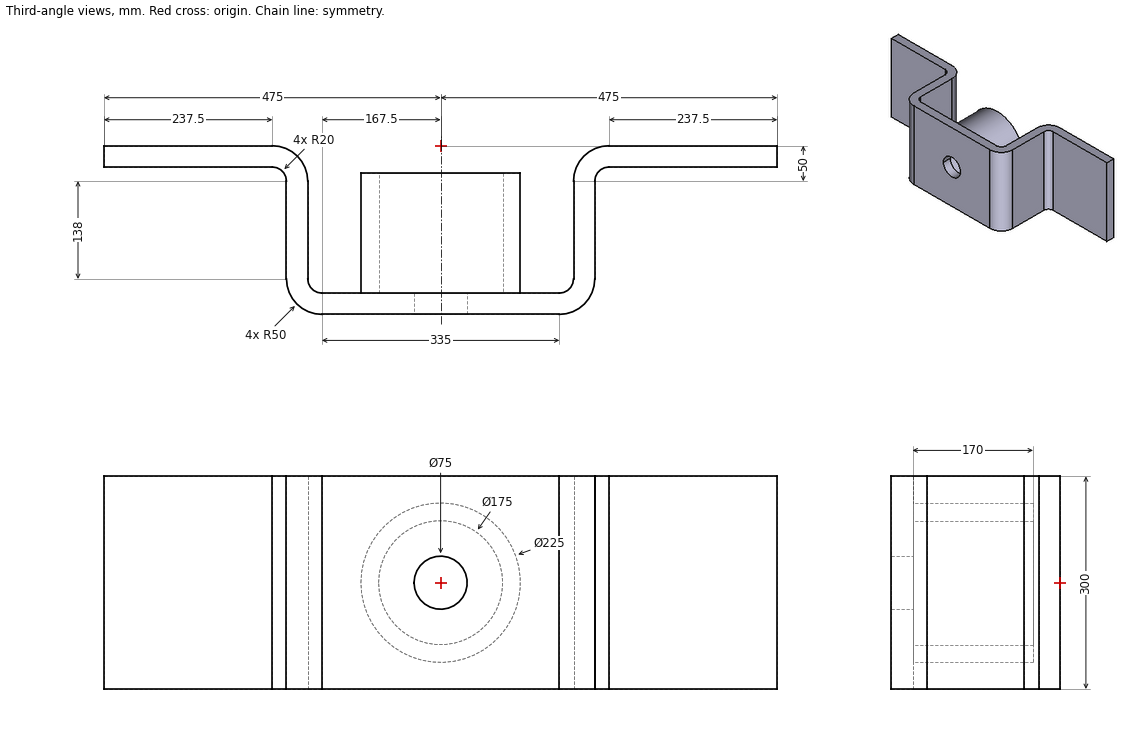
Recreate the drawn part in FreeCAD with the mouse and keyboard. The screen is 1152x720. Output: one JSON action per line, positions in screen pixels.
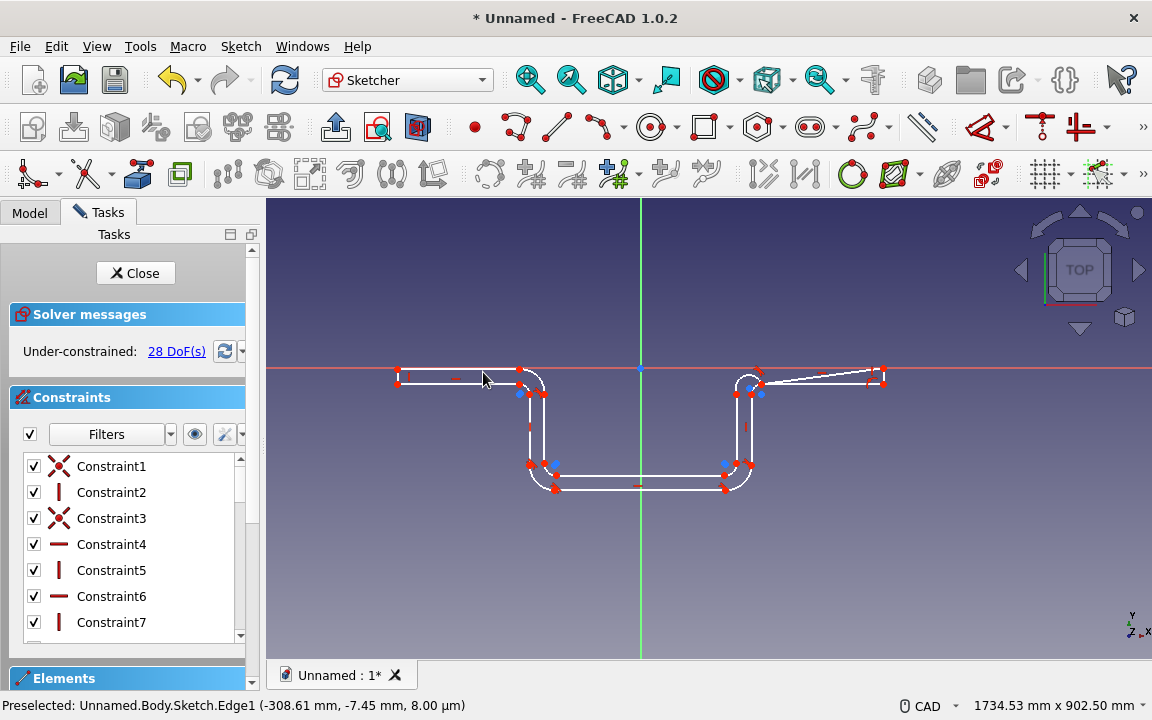
{"action": "scroll", "coordinate": [847, 373], "scroll_direction": "up", "scroll_amount": 6}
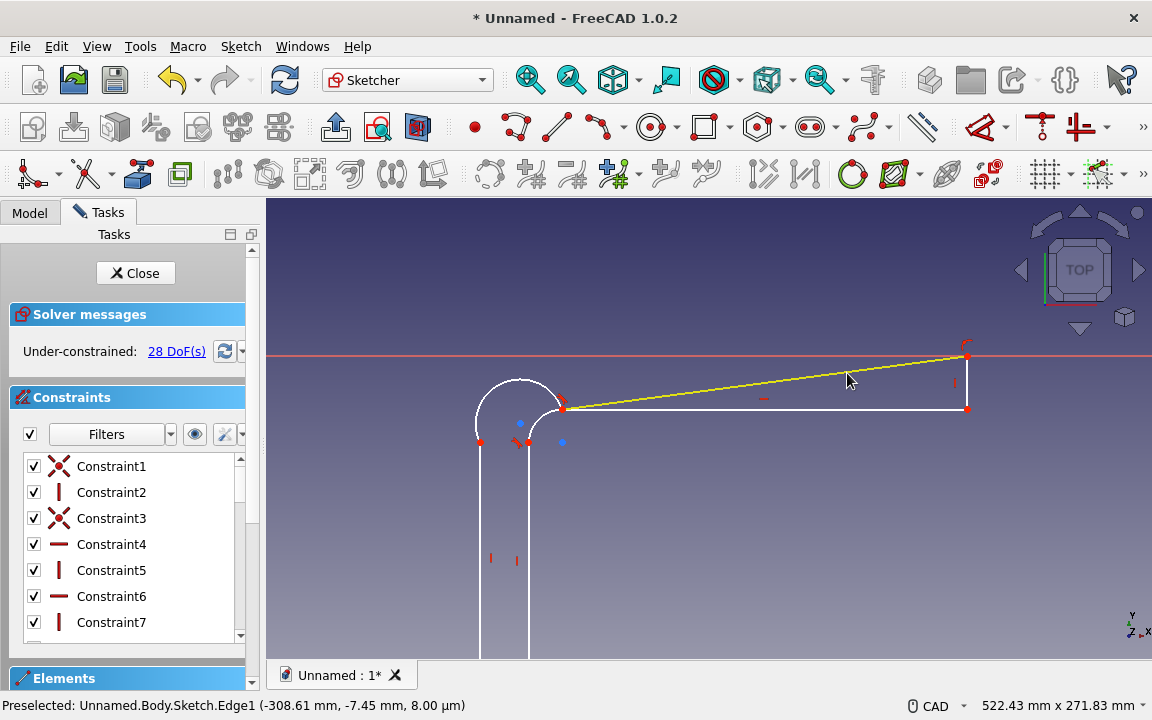
{"action": "left_click", "coordinate": [846, 372]}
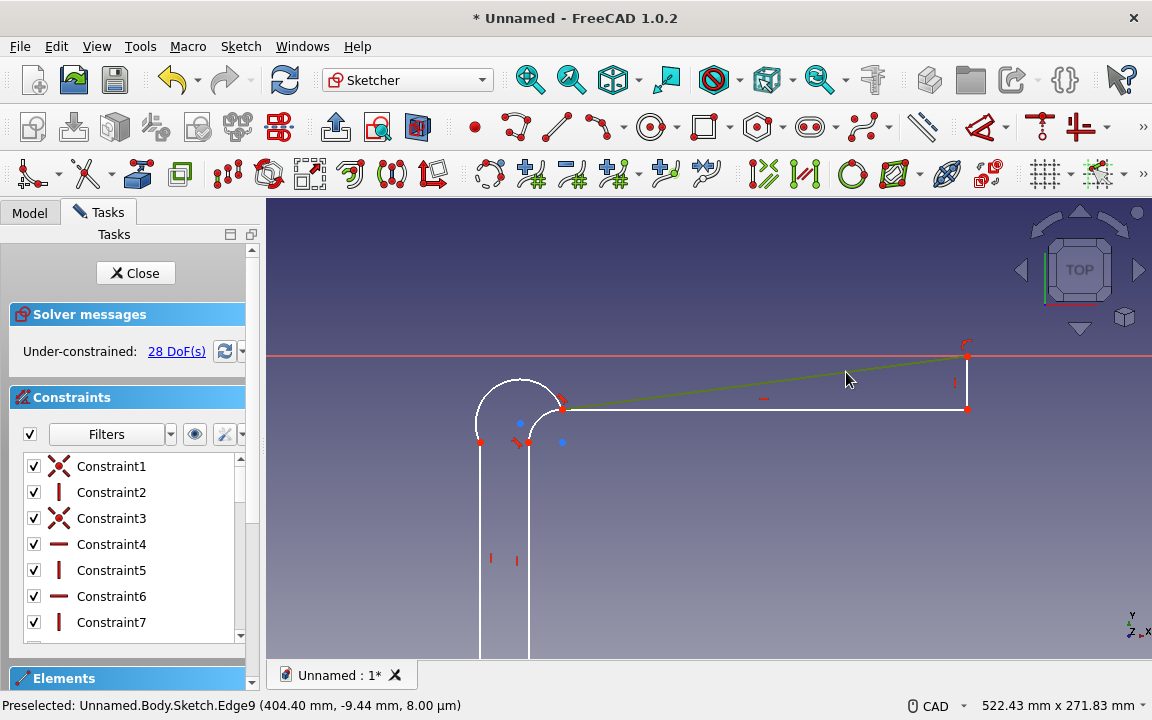
{"action": "key", "text": "h"}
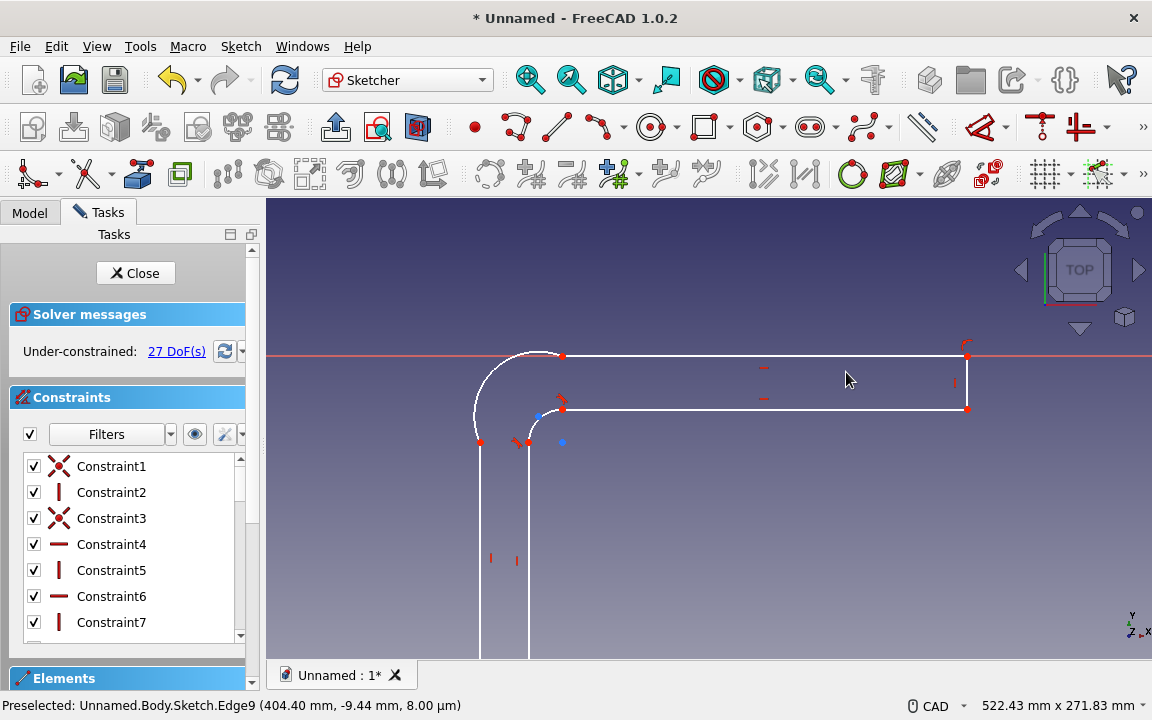
{"action": "left_click", "coordinate": [547, 413]}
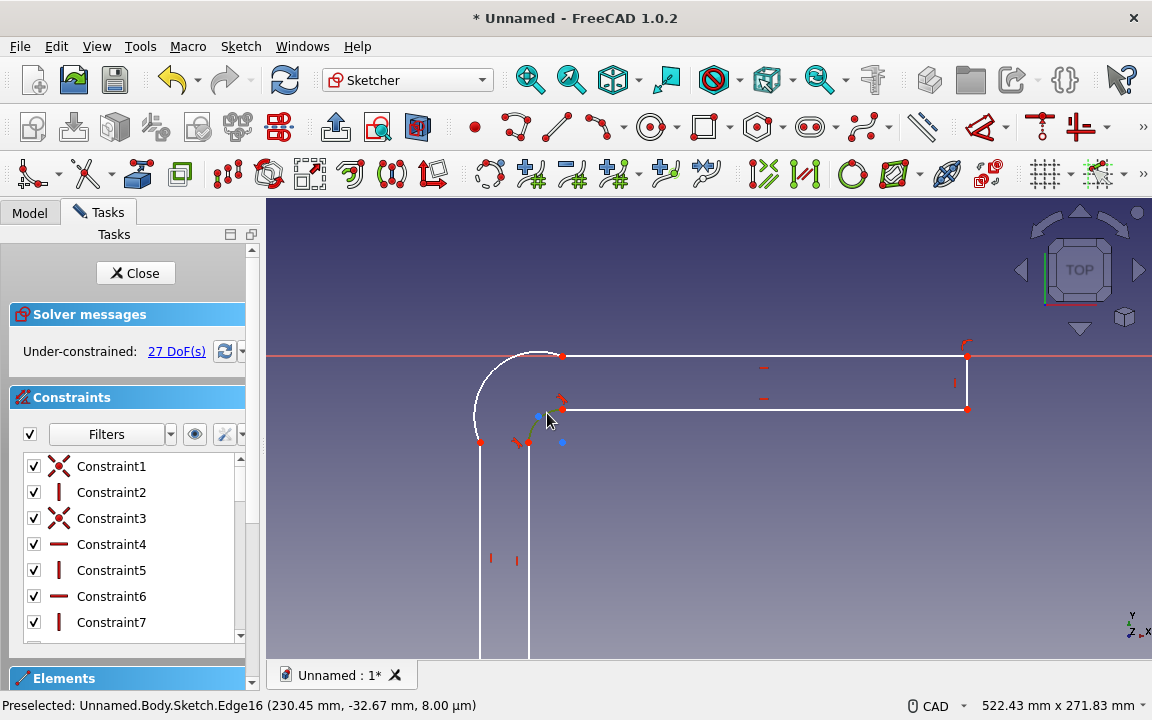
{"action": "left_click", "coordinate": [517, 356]}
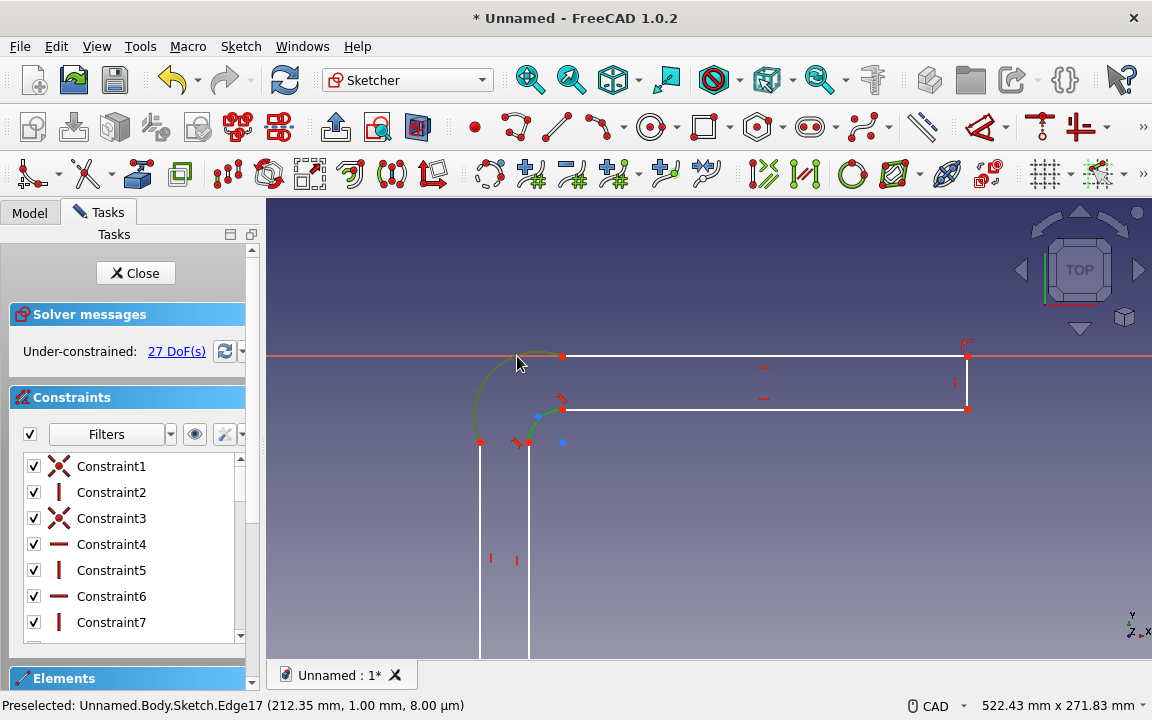
{"action": "key", "text": "c"}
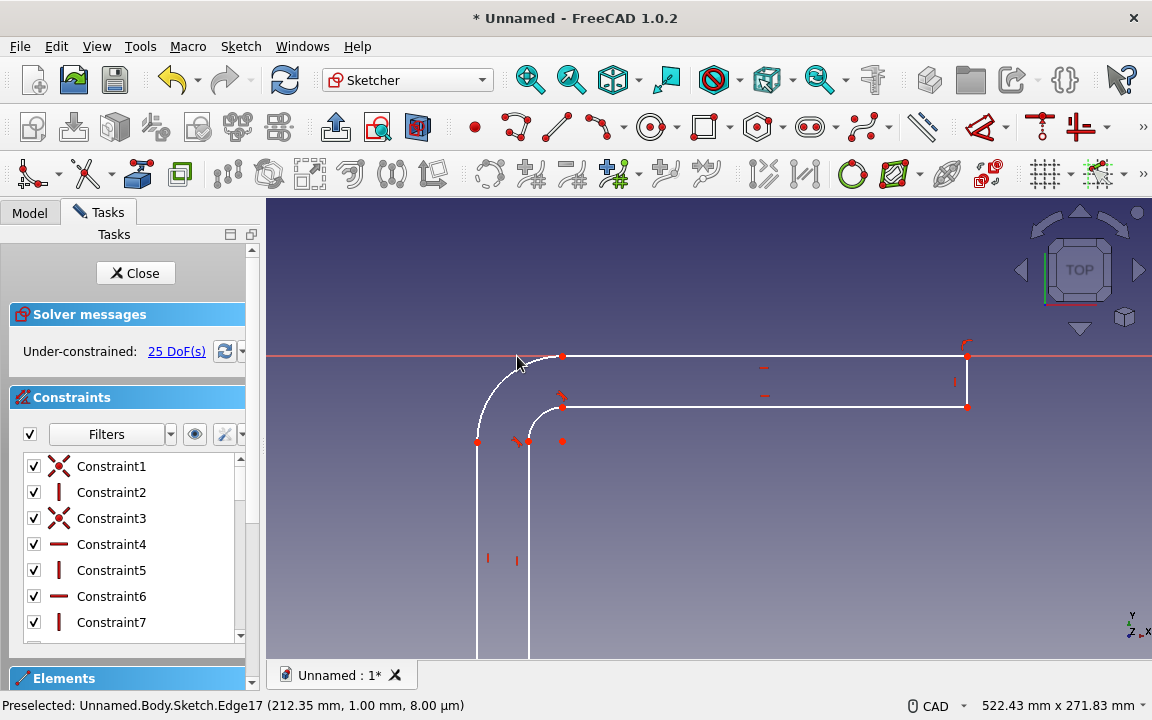
{"action": "scroll", "coordinate": [848, 373], "scroll_direction": "down", "scroll_amount": 6}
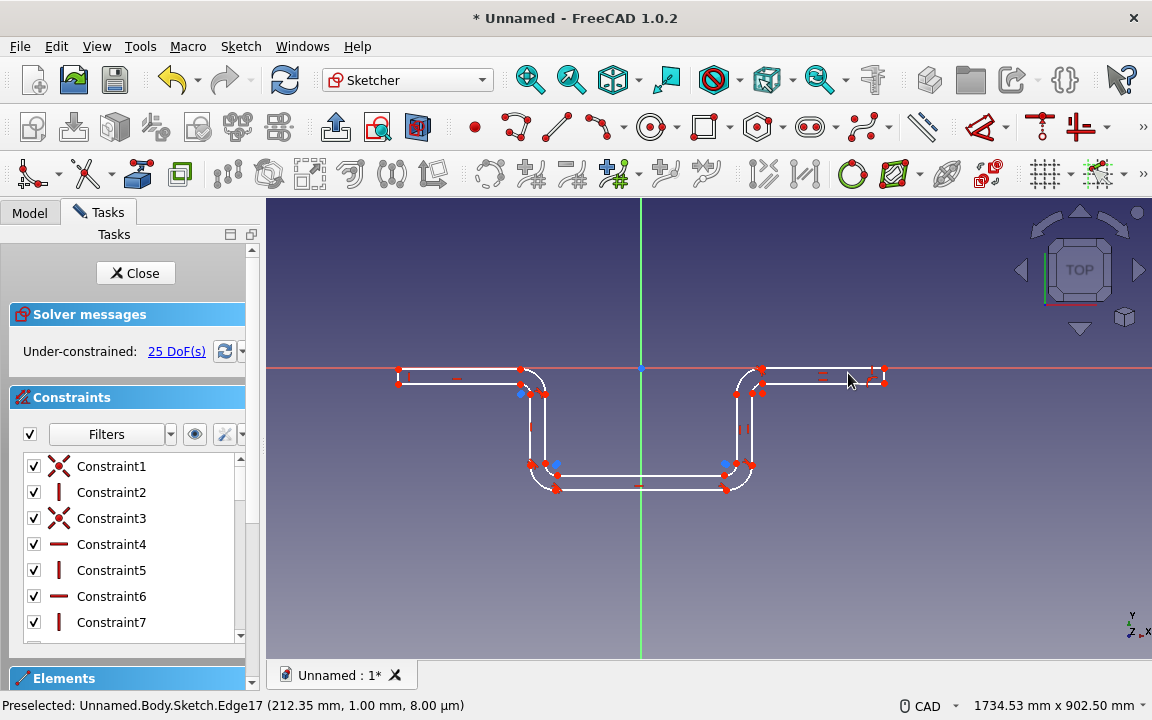
{"action": "left_click", "coordinate": [738, 487]}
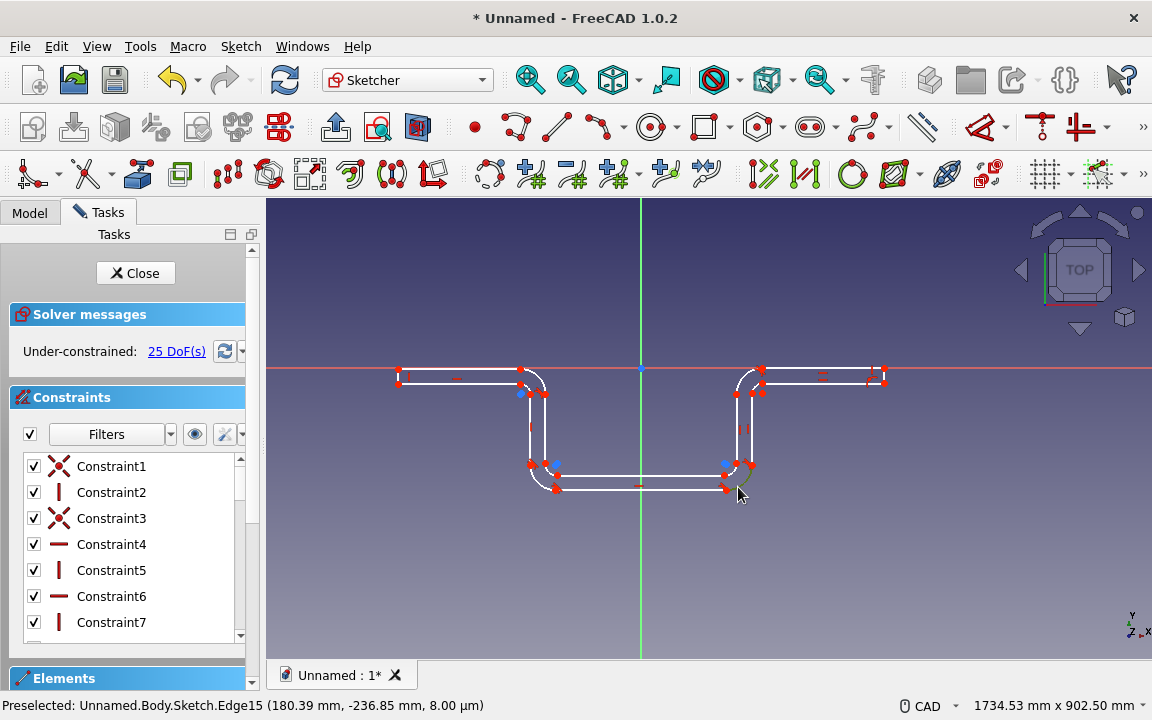
{"action": "scroll", "coordinate": [733, 472], "scroll_direction": "up", "scroll_amount": 2}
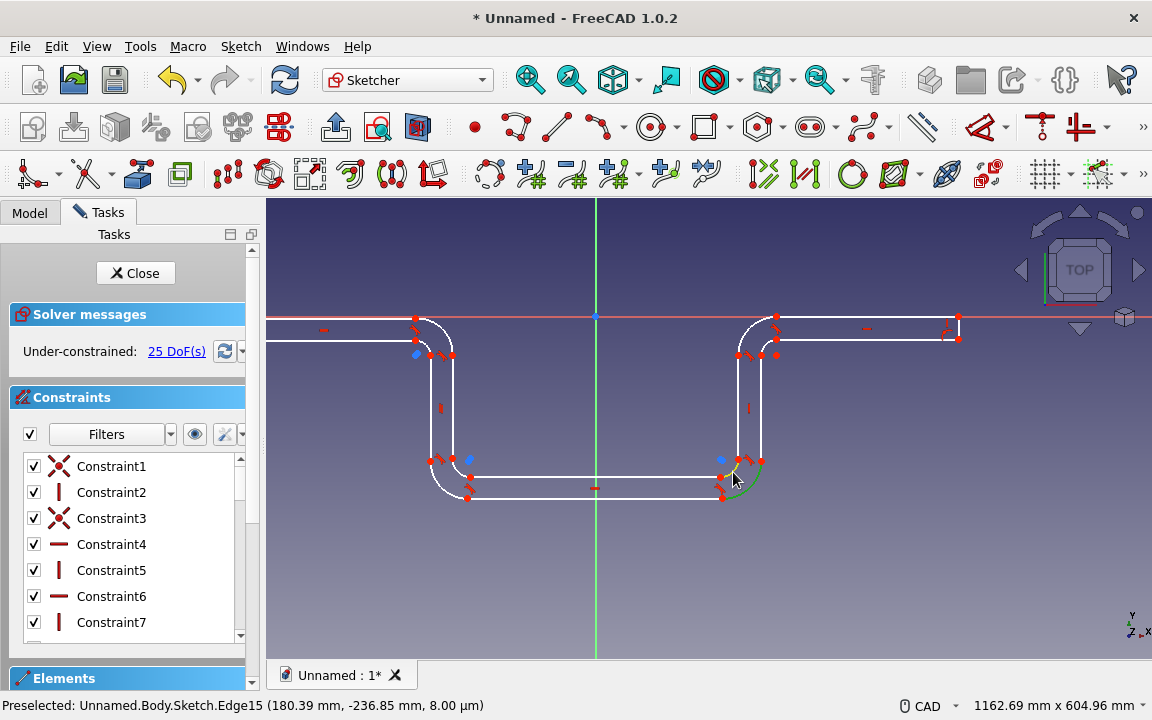
{"action": "left_click", "coordinate": [733, 472]}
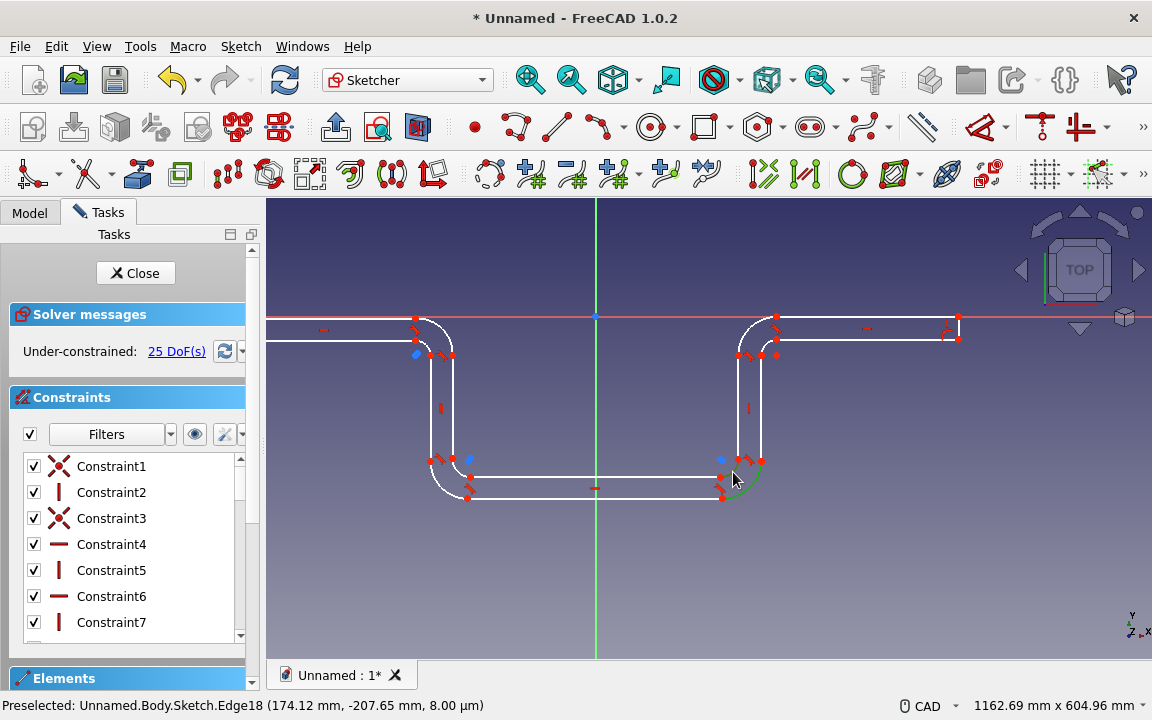
{"action": "key", "text": "c"}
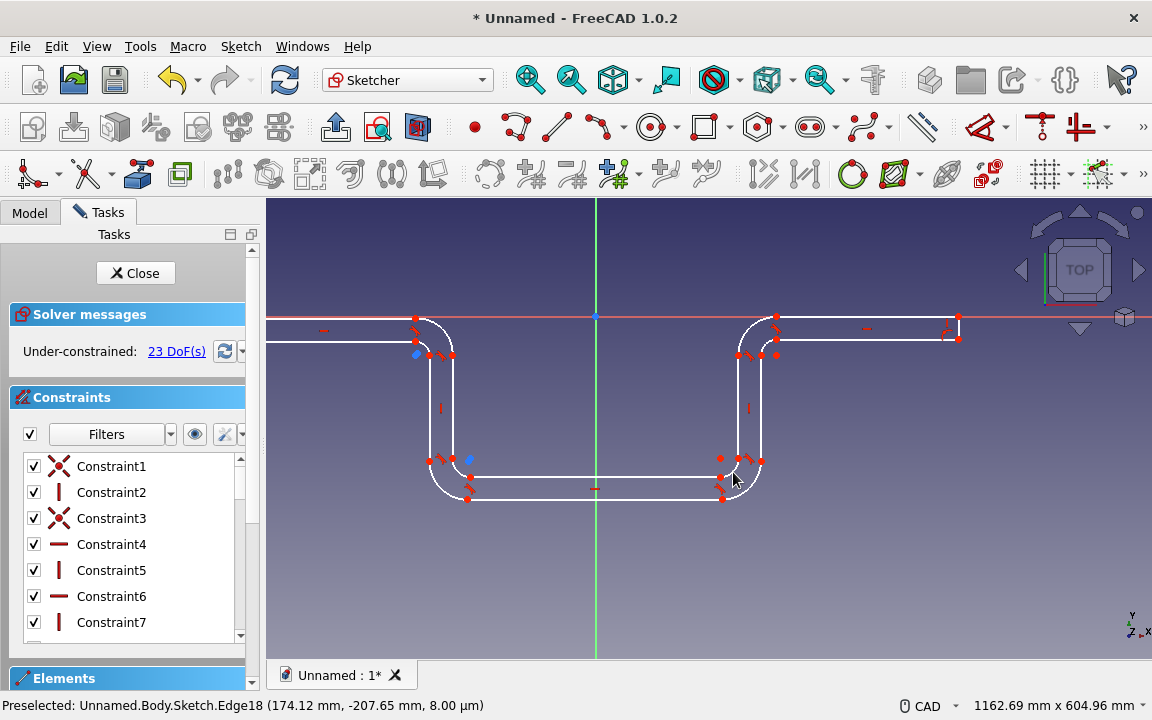
{"action": "left_click", "coordinate": [434, 479]}